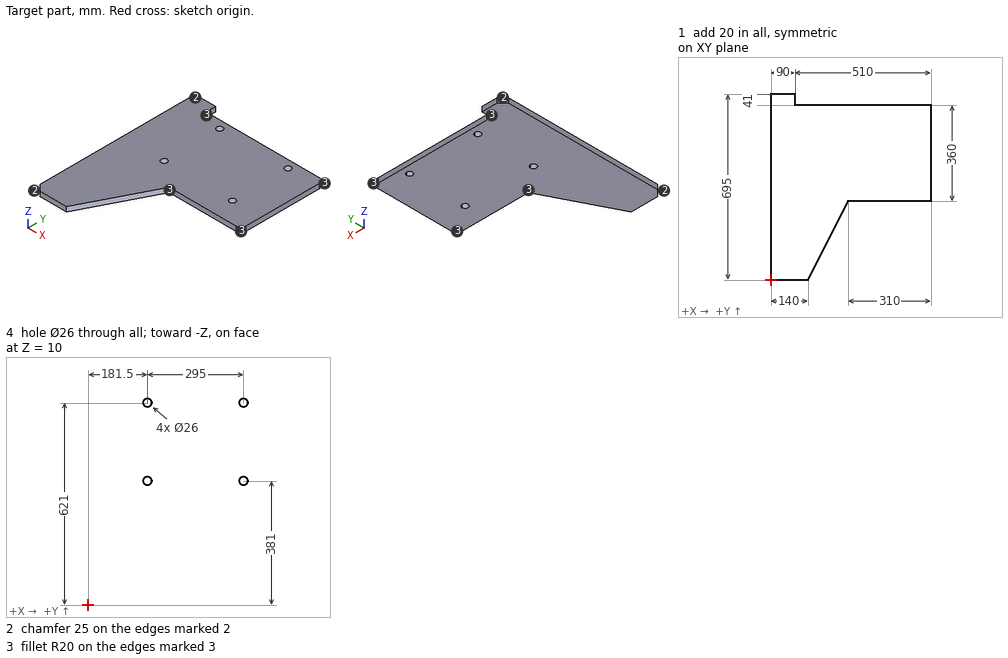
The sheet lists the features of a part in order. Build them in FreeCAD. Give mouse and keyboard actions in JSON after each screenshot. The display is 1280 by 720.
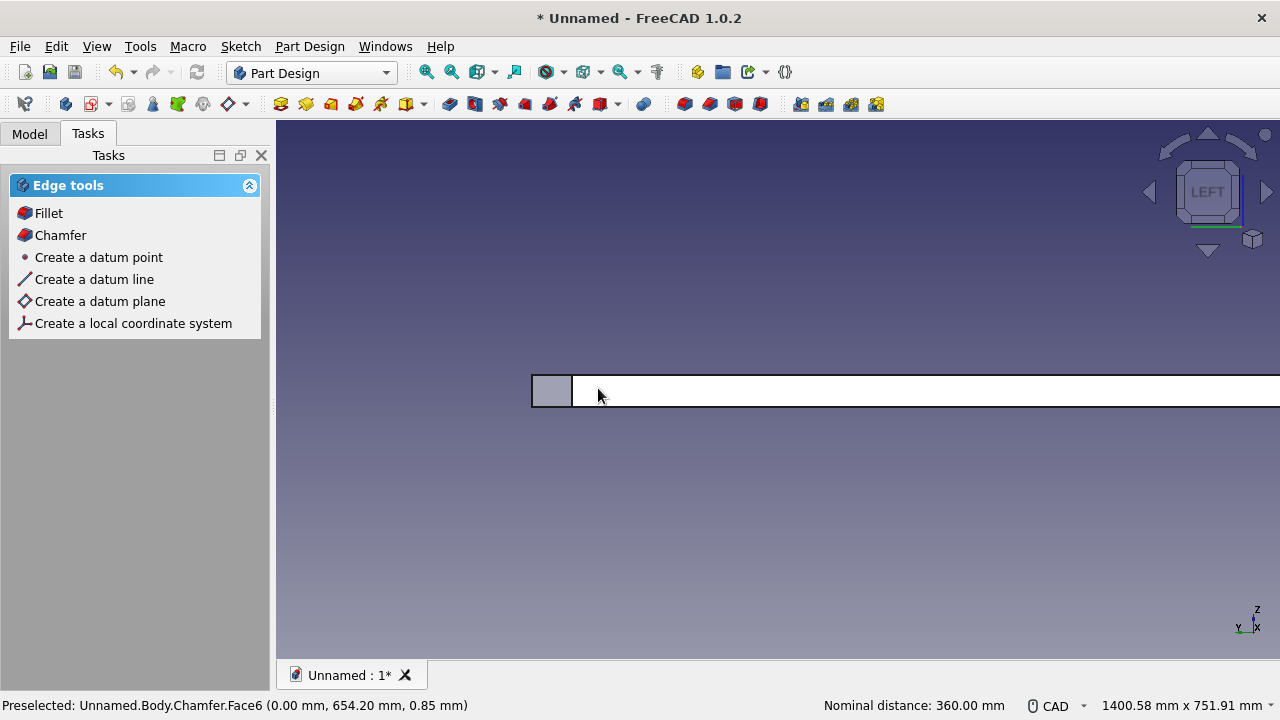
{"action": "left_click", "coordinate": [427, 72]}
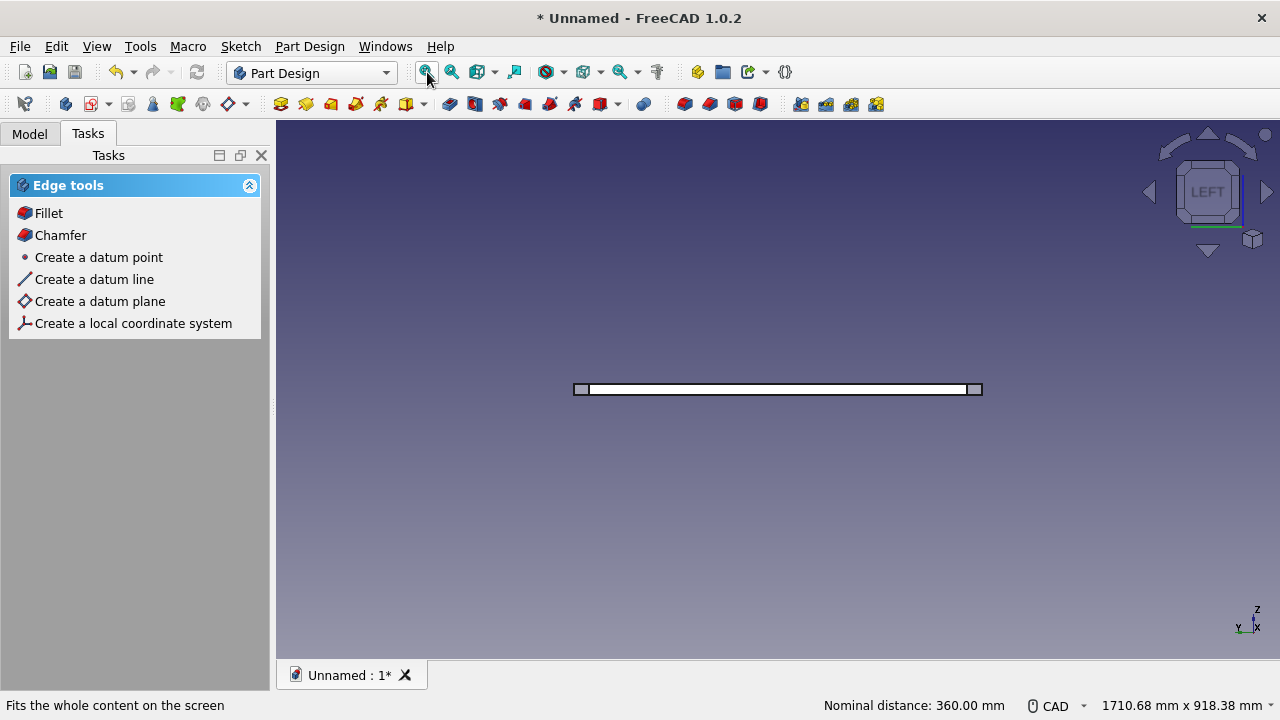
{"action": "key", "text": "v 3"}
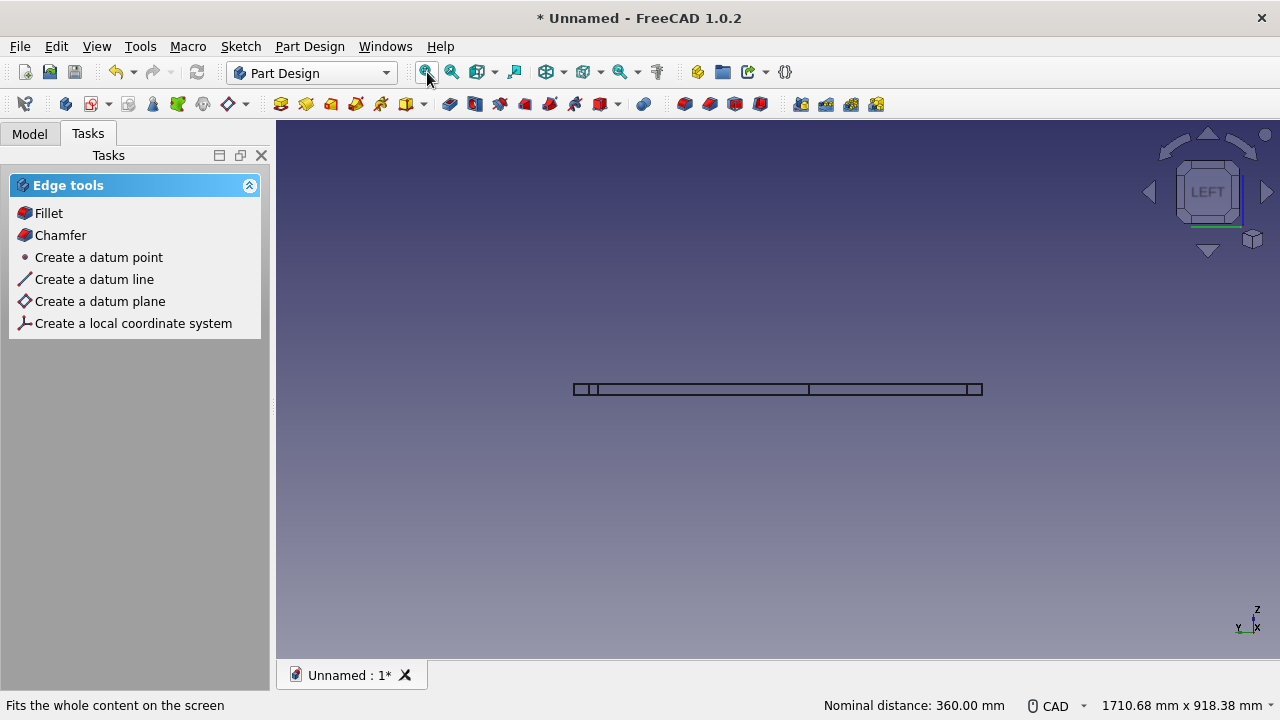
{"action": "key", "text": "0"}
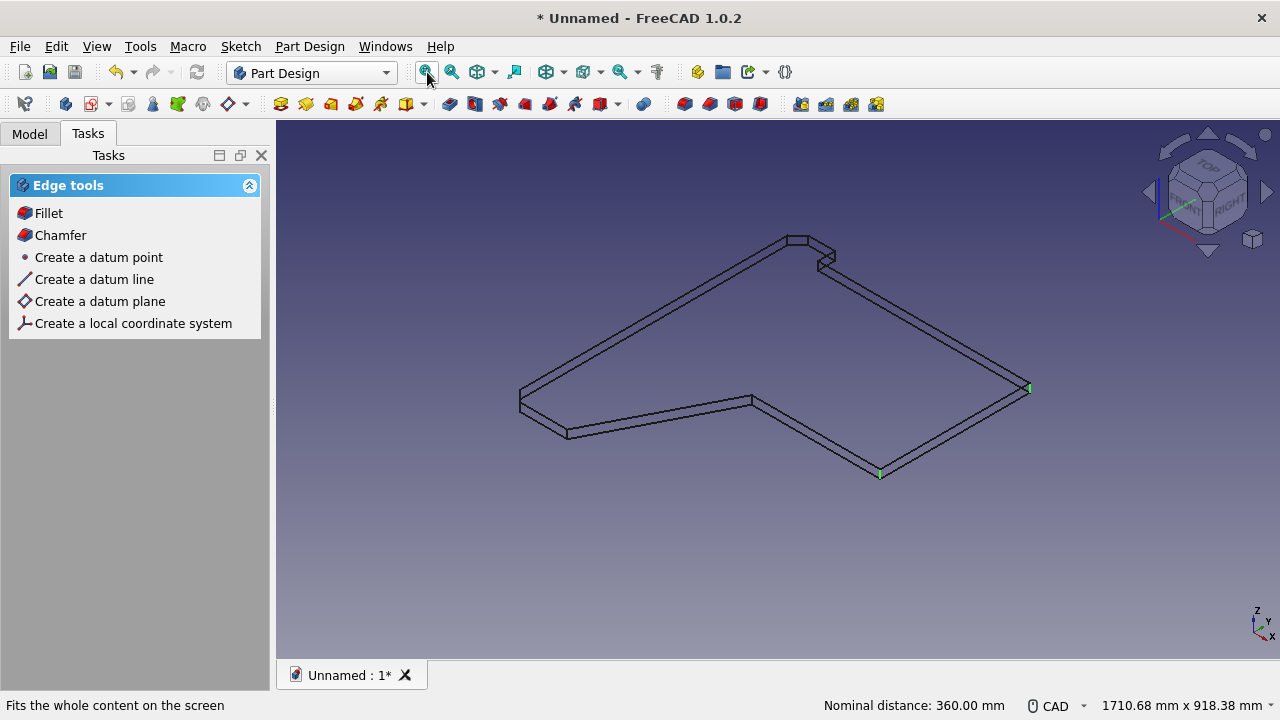
{"action": "scroll", "coordinate": [818, 265], "scroll_direction": "up", "scroll_amount": 7}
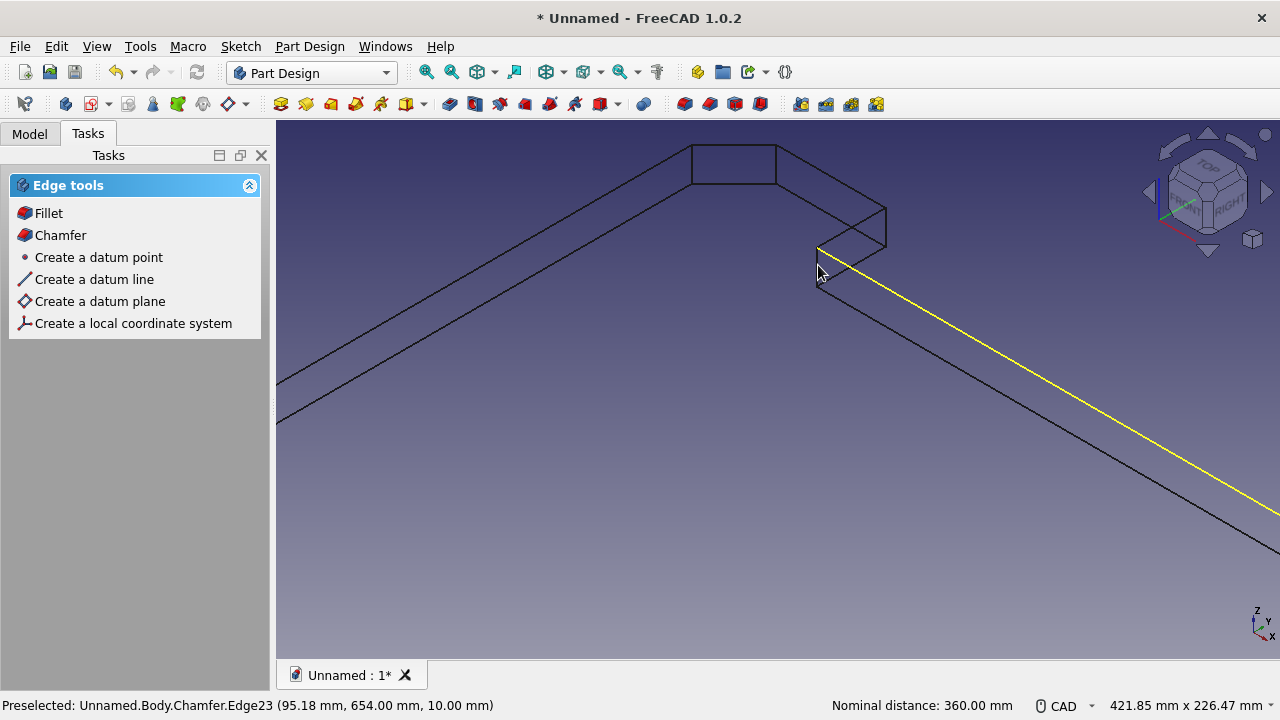
{"action": "left_click", "coordinate": [817, 266], "text": "ctrl"}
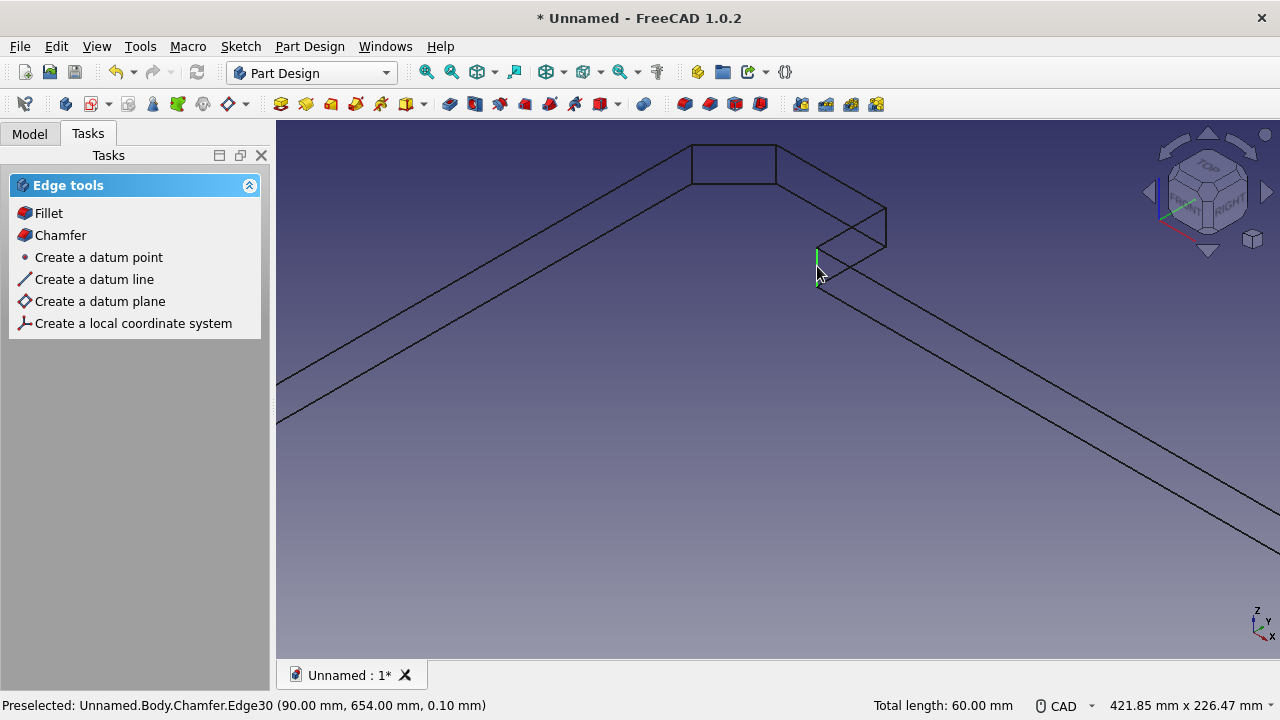
{"action": "left_click", "coordinate": [427, 72]}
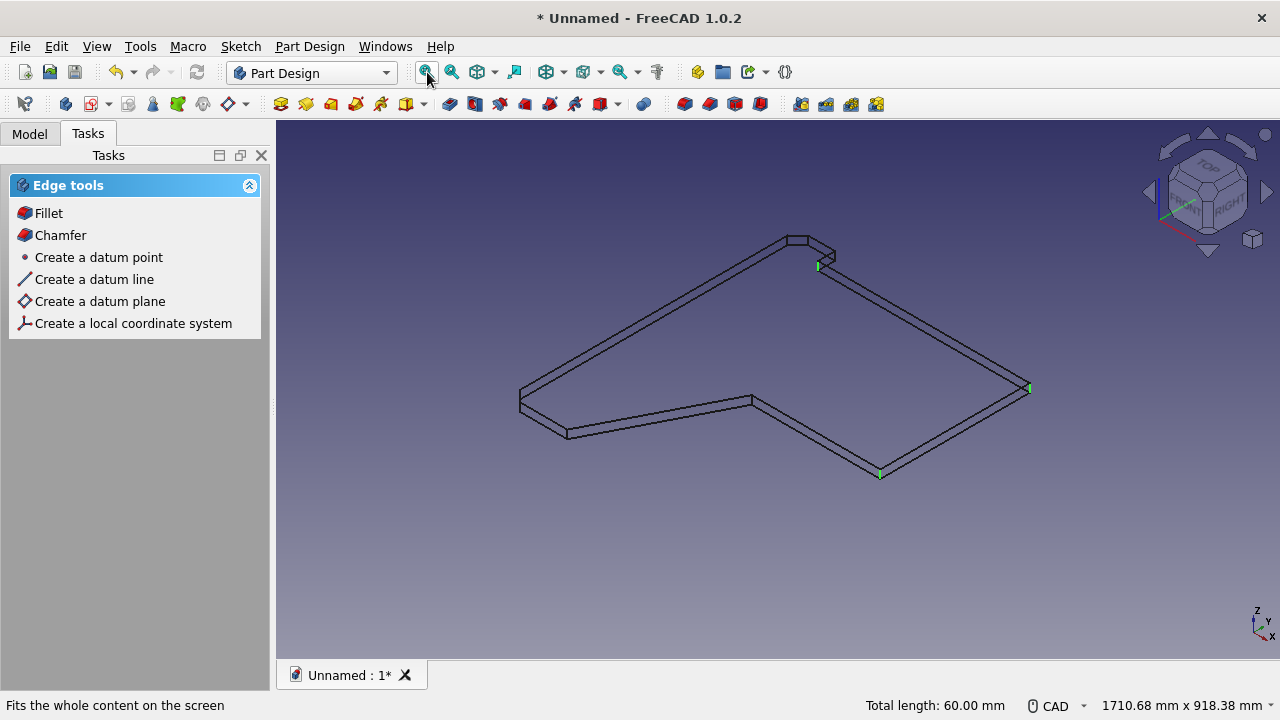
{"action": "key", "text": "2"}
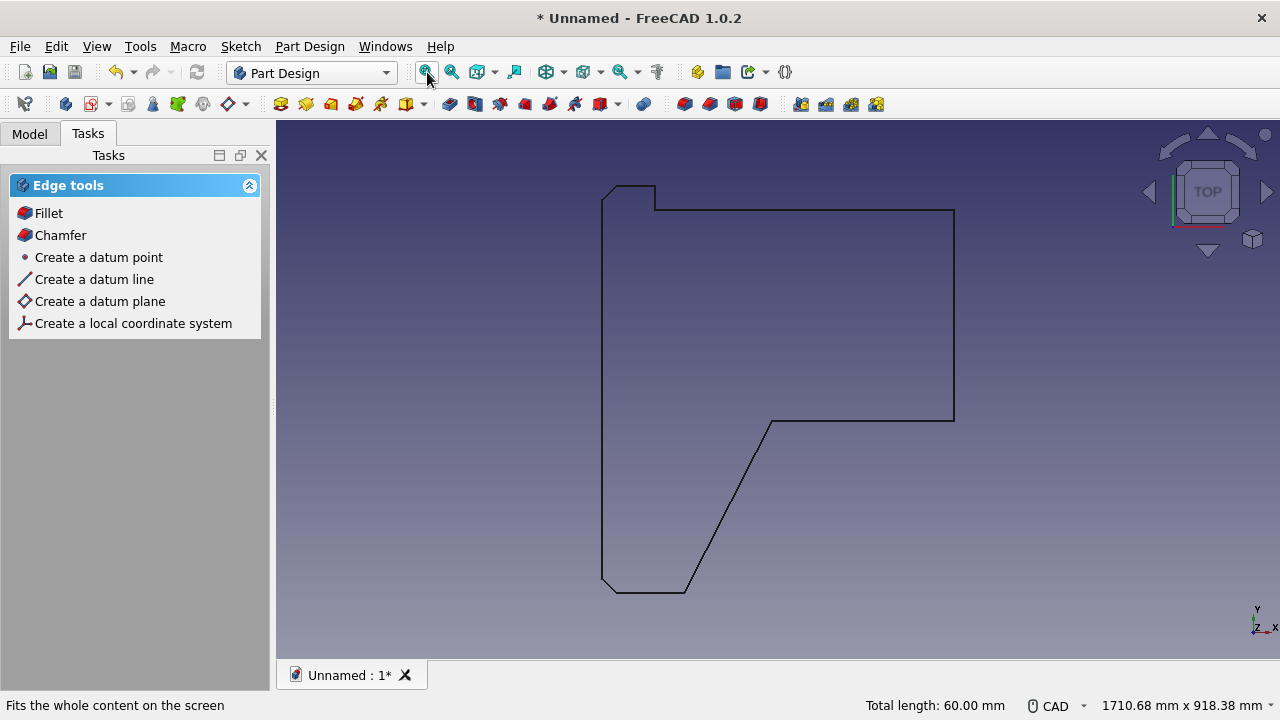
{"action": "scroll", "coordinate": [772, 420], "scroll_direction": "up", "scroll_amount": 7}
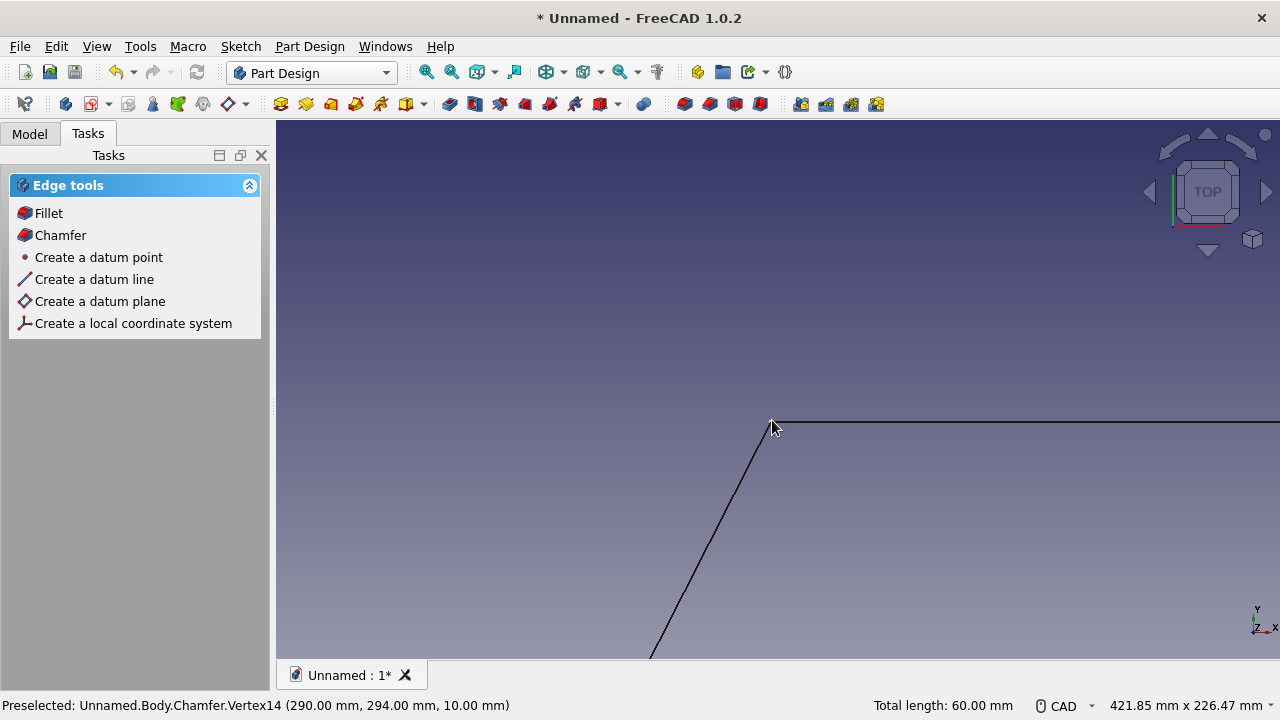
{"action": "left_click", "coordinate": [427, 72]}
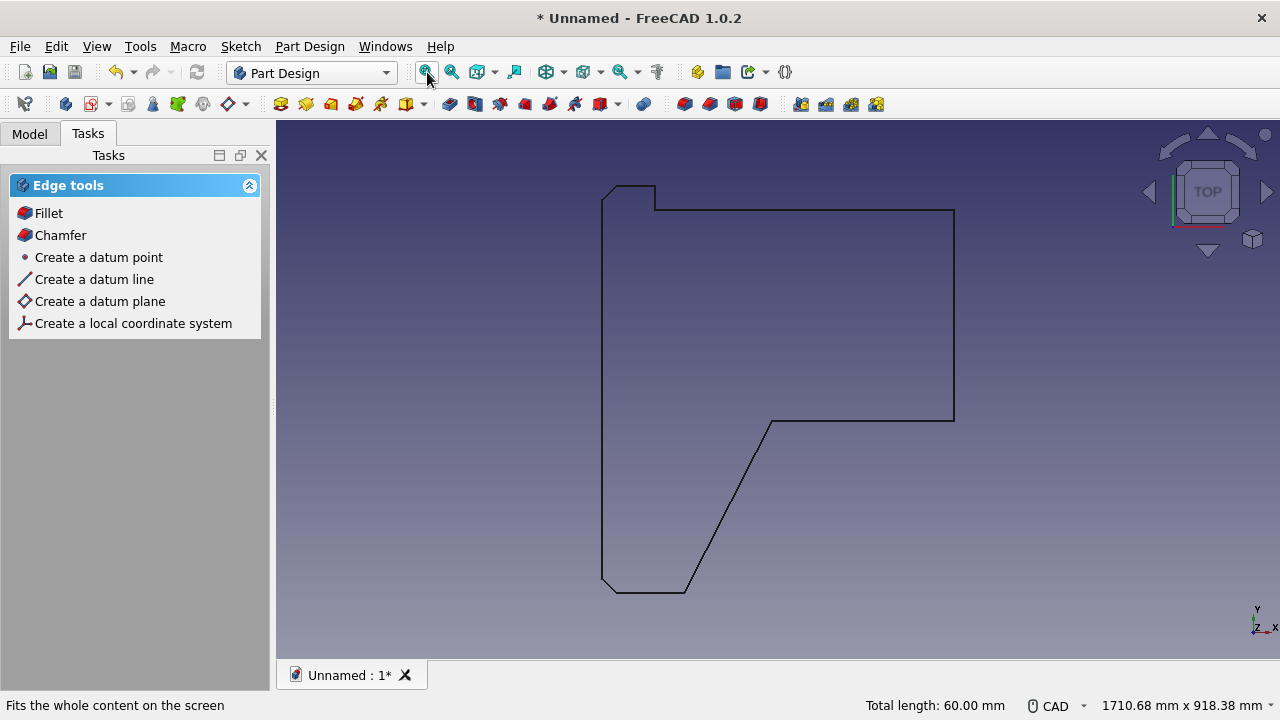
{"action": "key", "text": "1"}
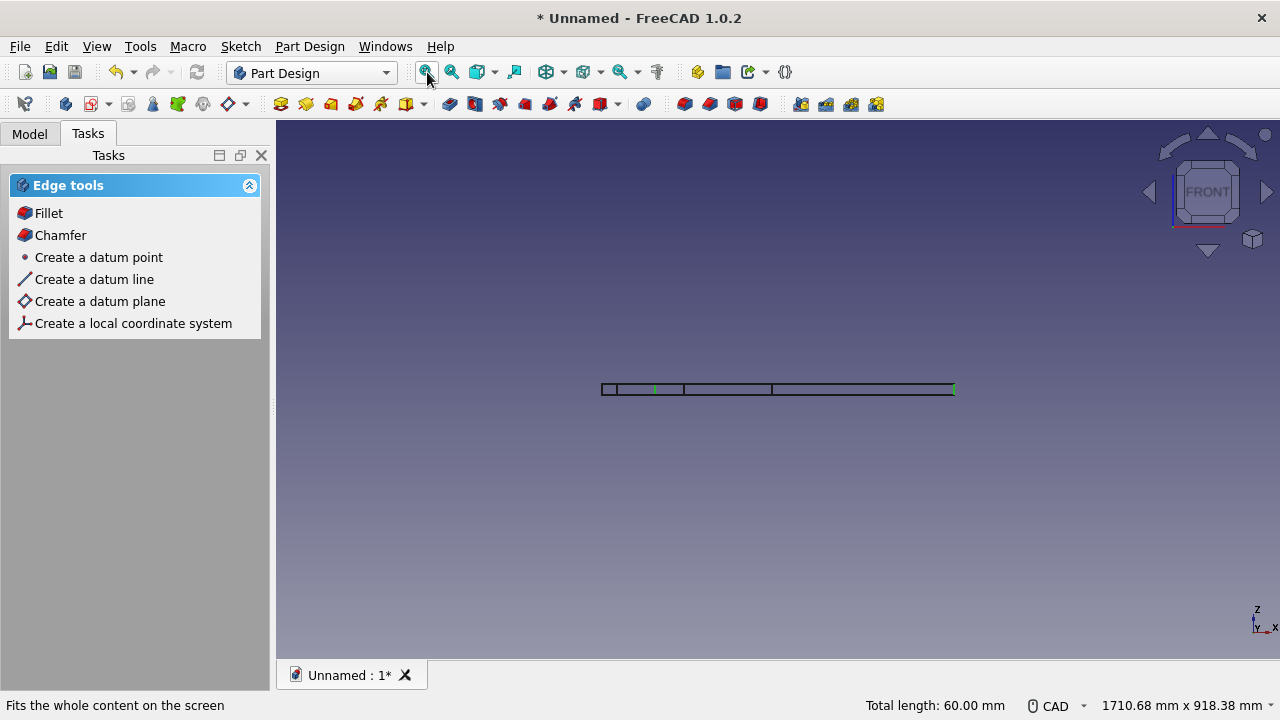
{"action": "left_click", "coordinate": [427, 72]}